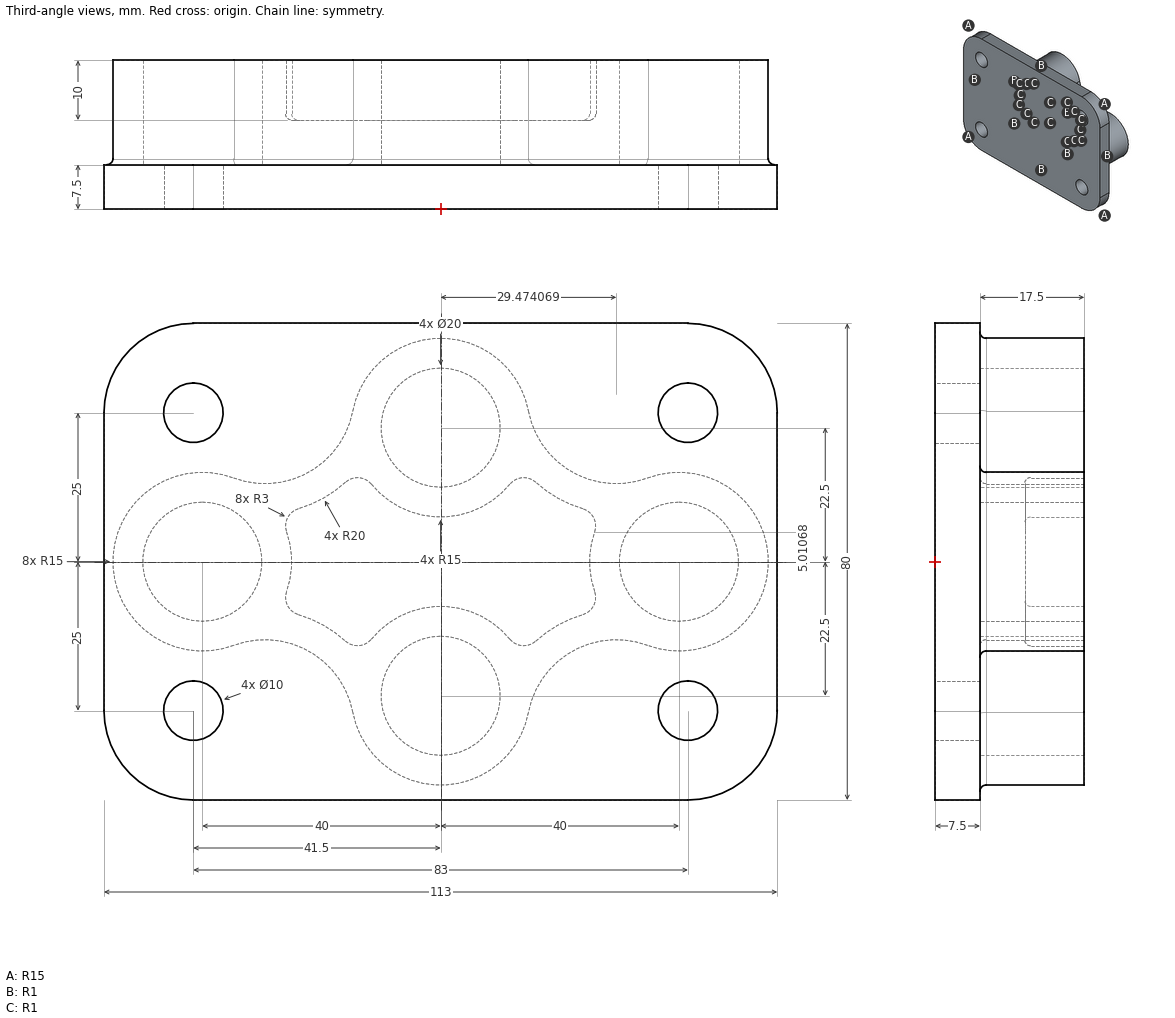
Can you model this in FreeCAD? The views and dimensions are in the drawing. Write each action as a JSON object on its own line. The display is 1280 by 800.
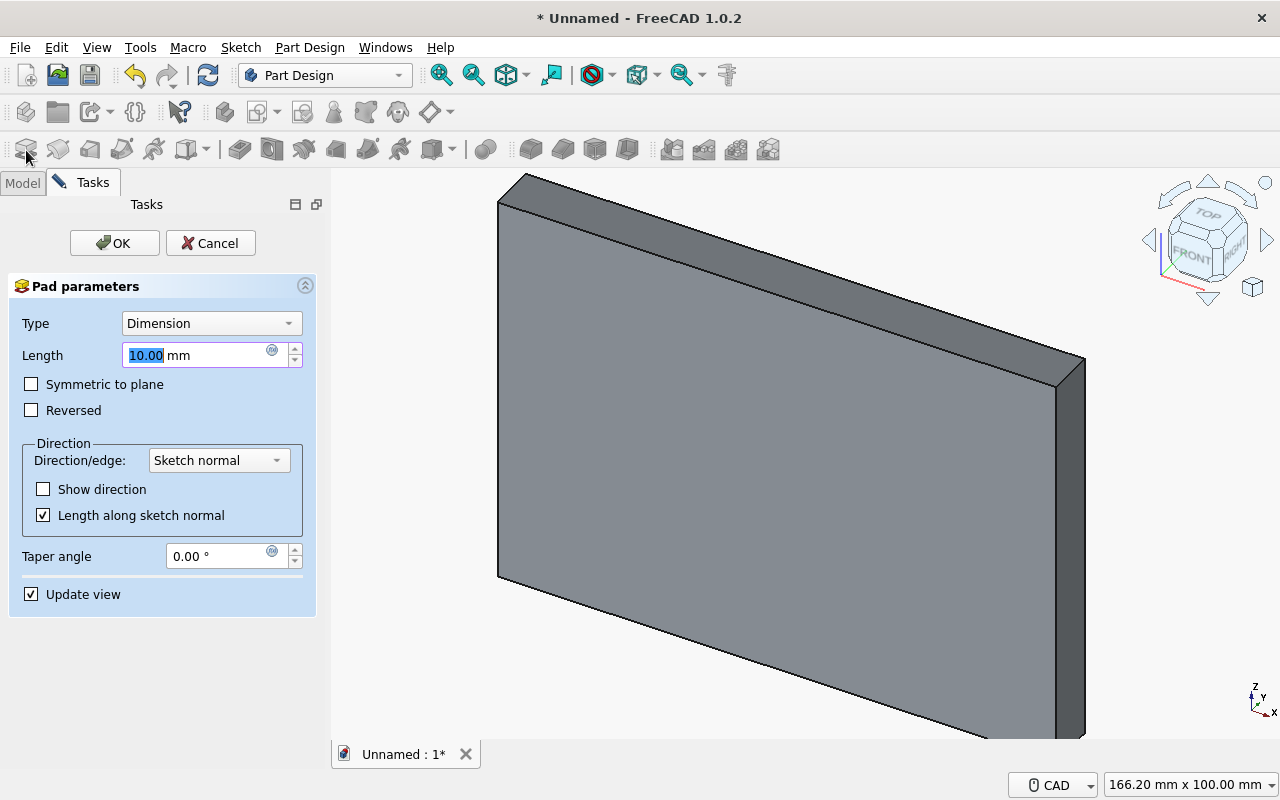
{"action": "type", "text": "7.5"}
{"action": "key", "text": "Tab"}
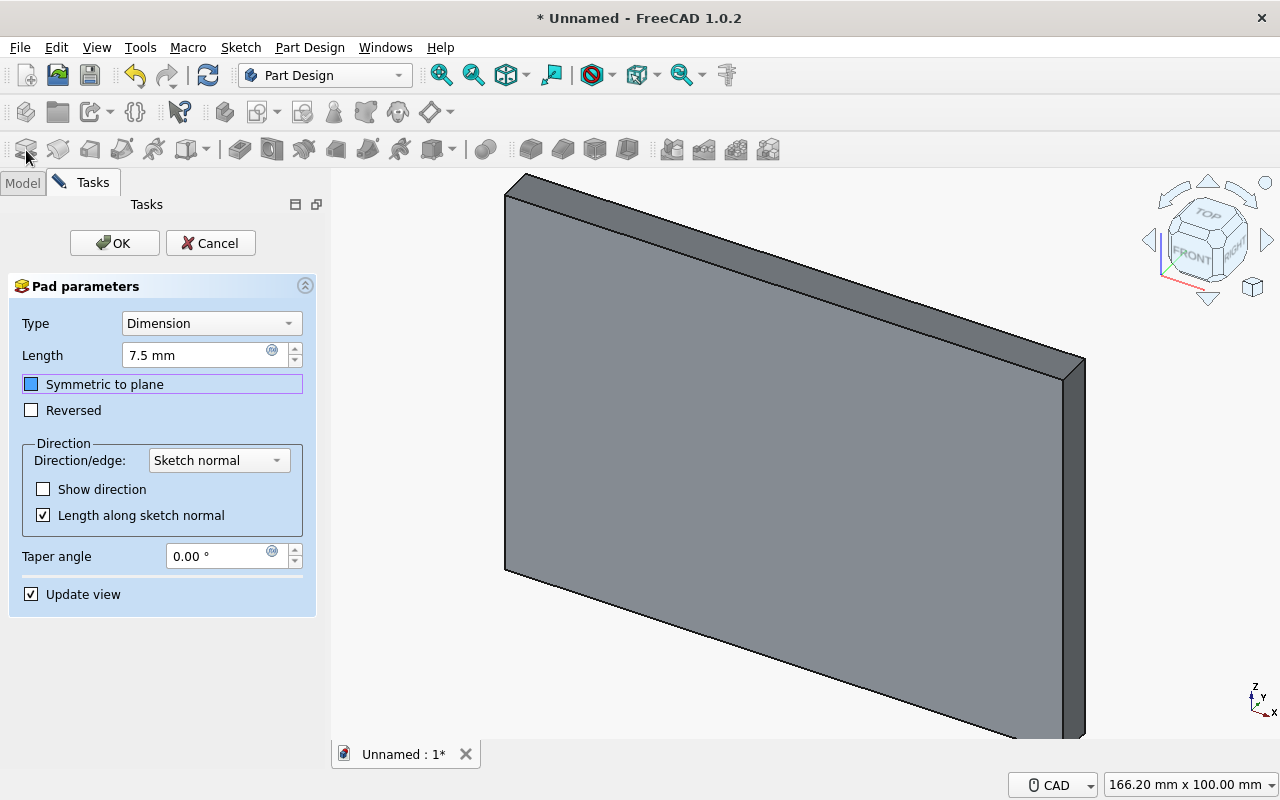
{"action": "left_click", "coordinate": [30, 410]}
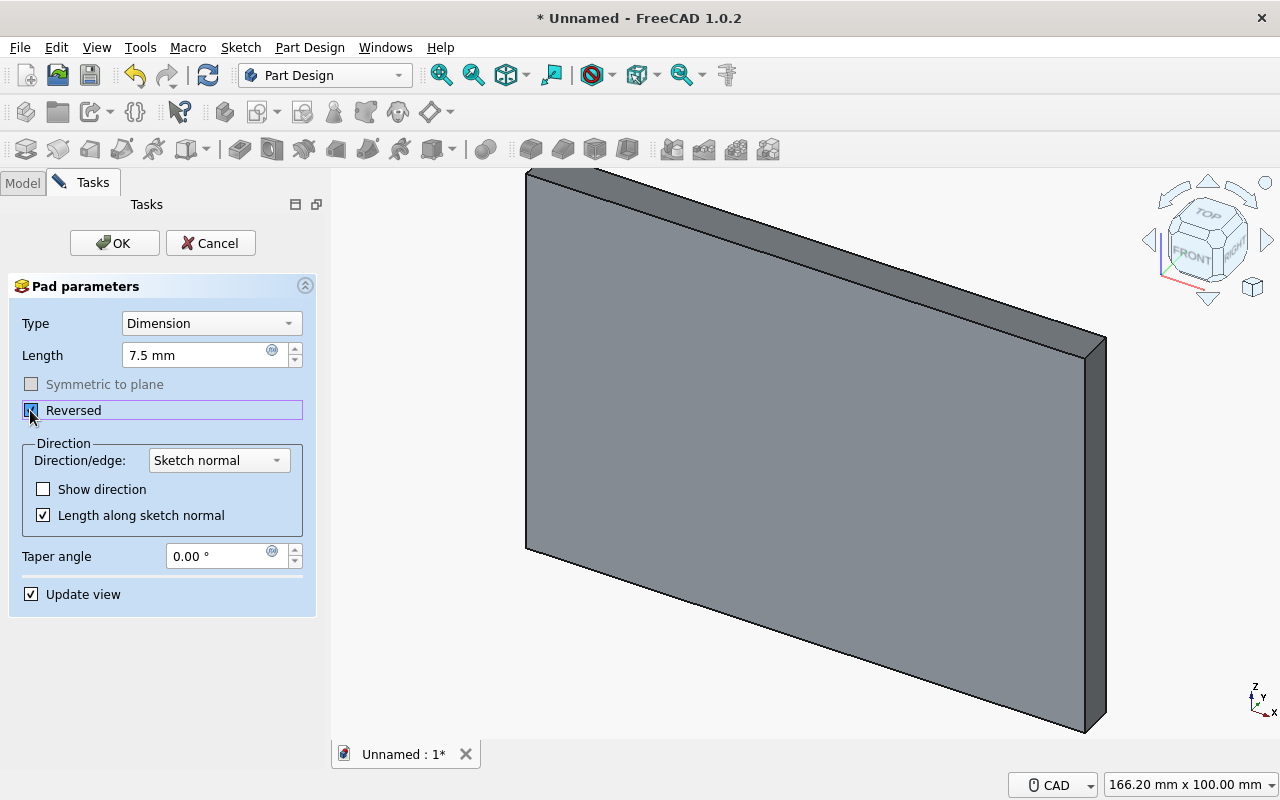
{"action": "left_click", "coordinate": [115, 243]}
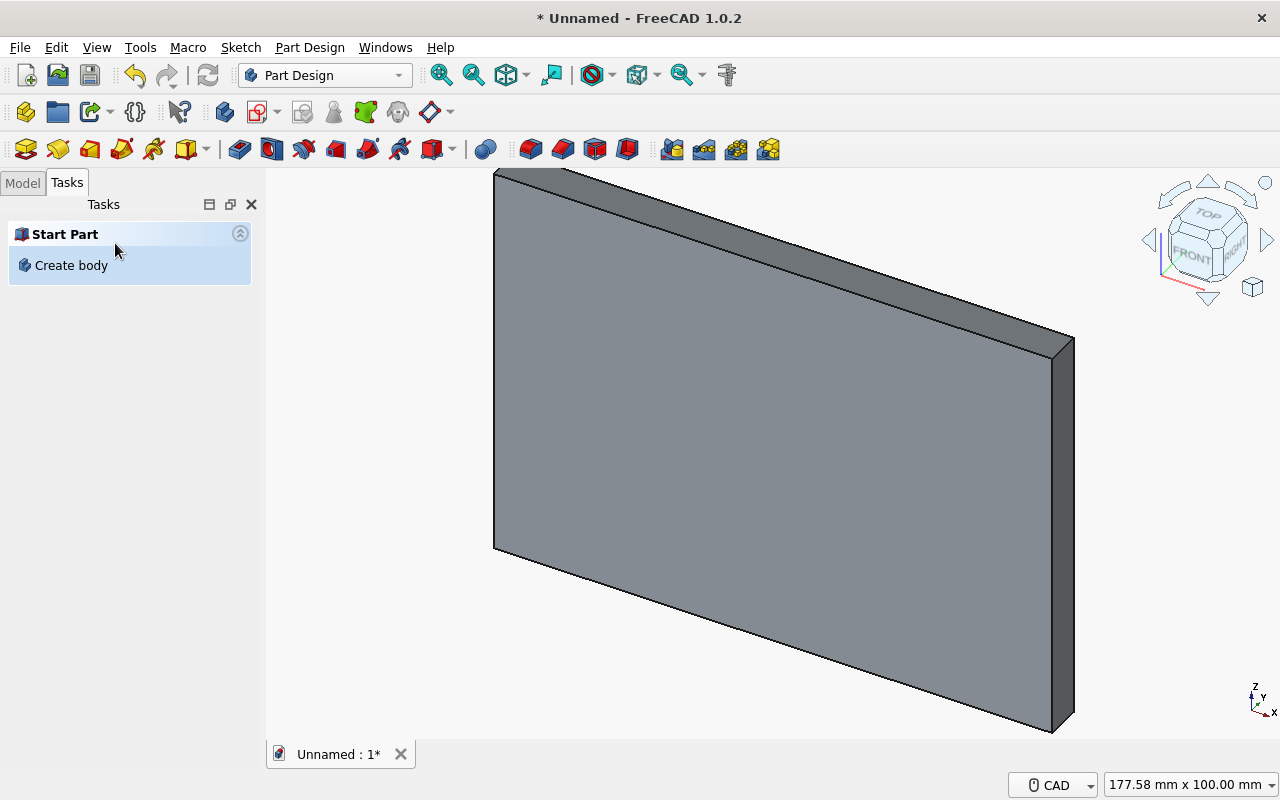
{"action": "left_click", "coordinate": [442, 76]}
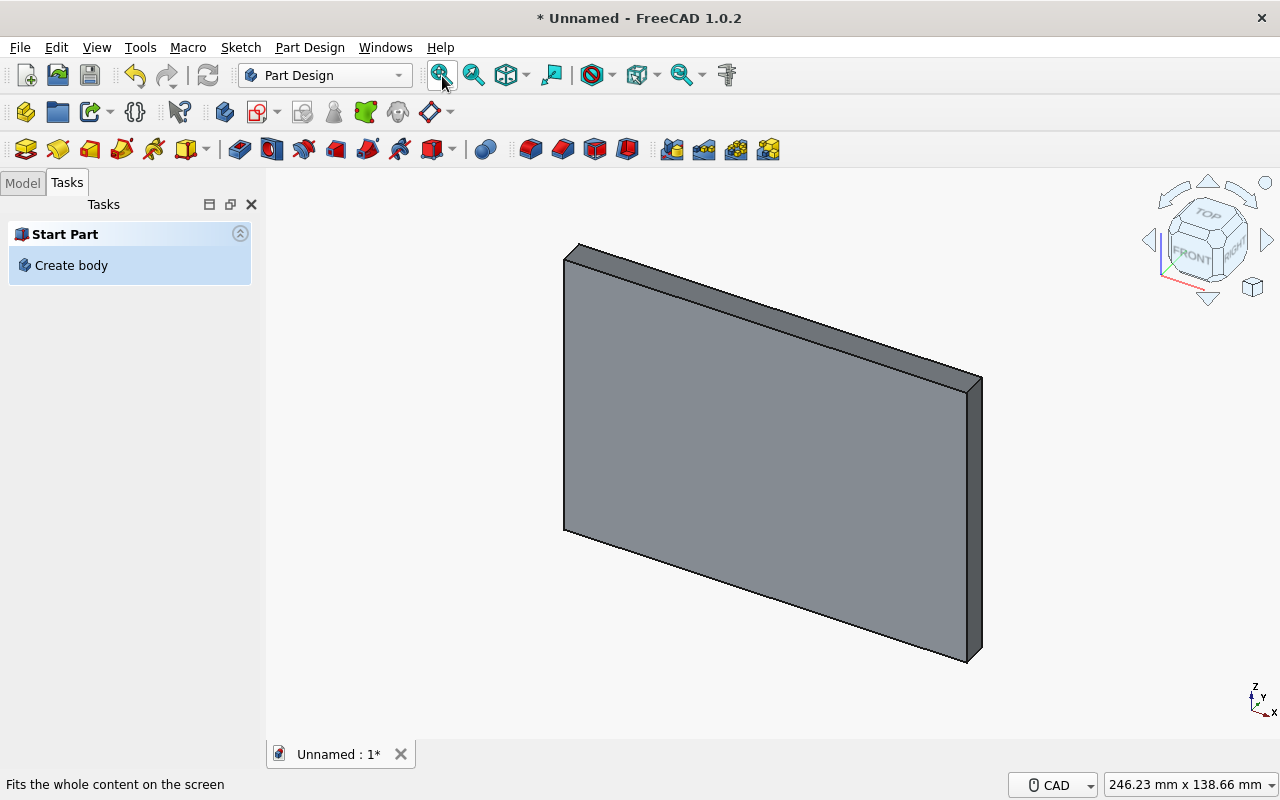
{"action": "left_click", "coordinate": [975, 384]}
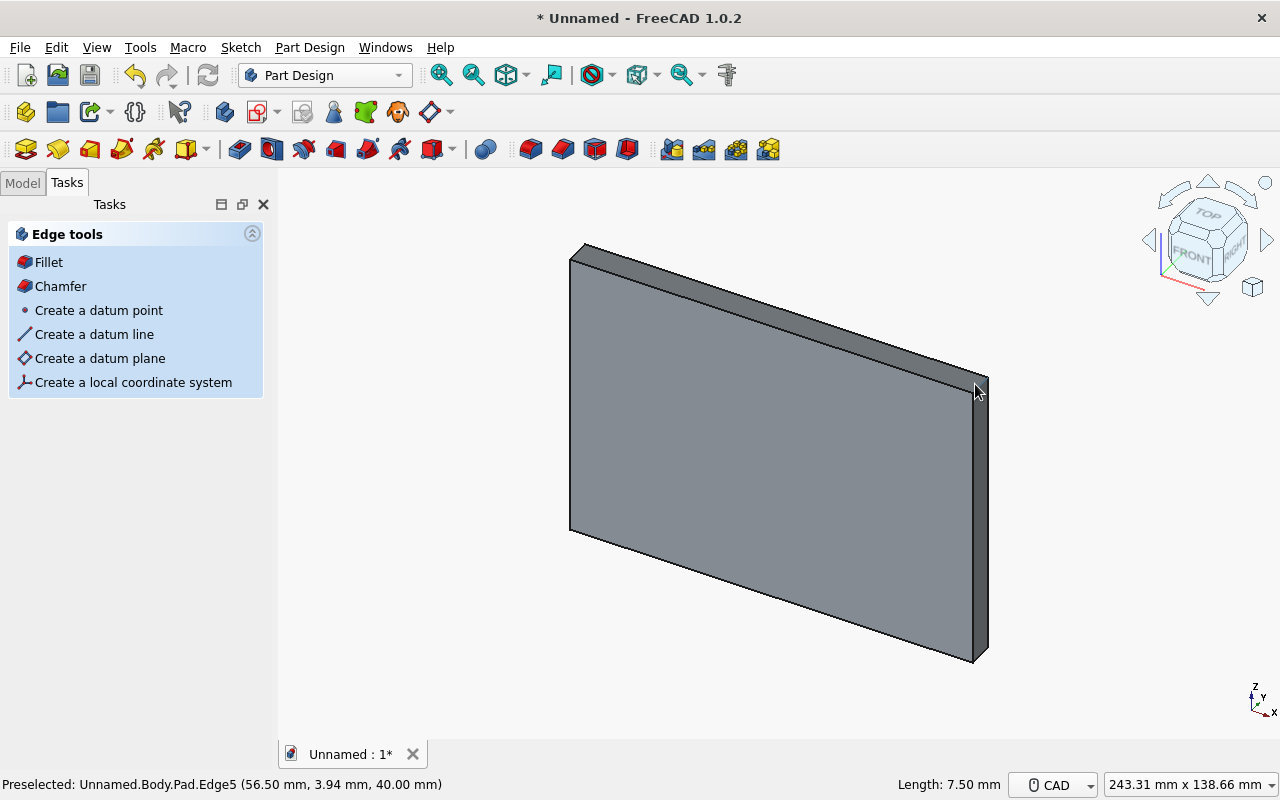
{"action": "key", "text": "0"}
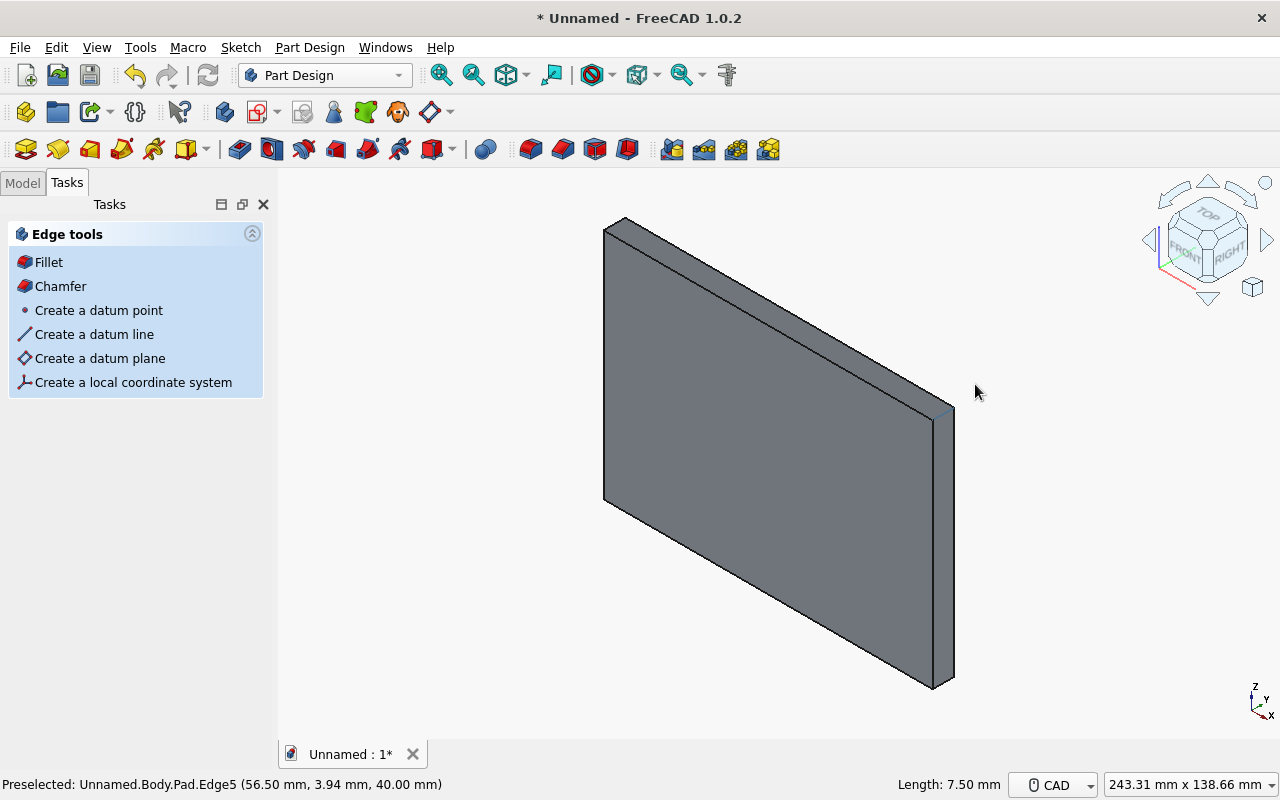
{"action": "key", "text": "2"}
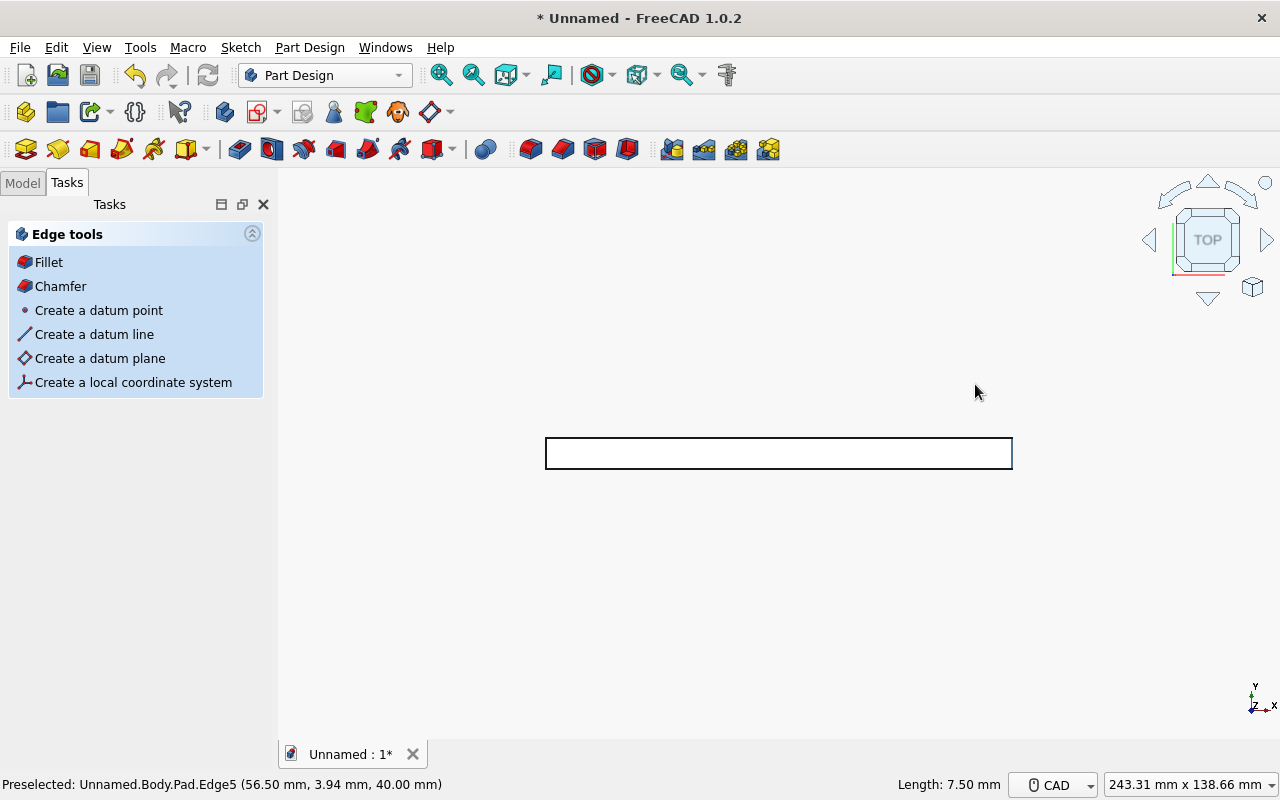
{"action": "left_click", "coordinate": [546, 453], "text": "ctrl"}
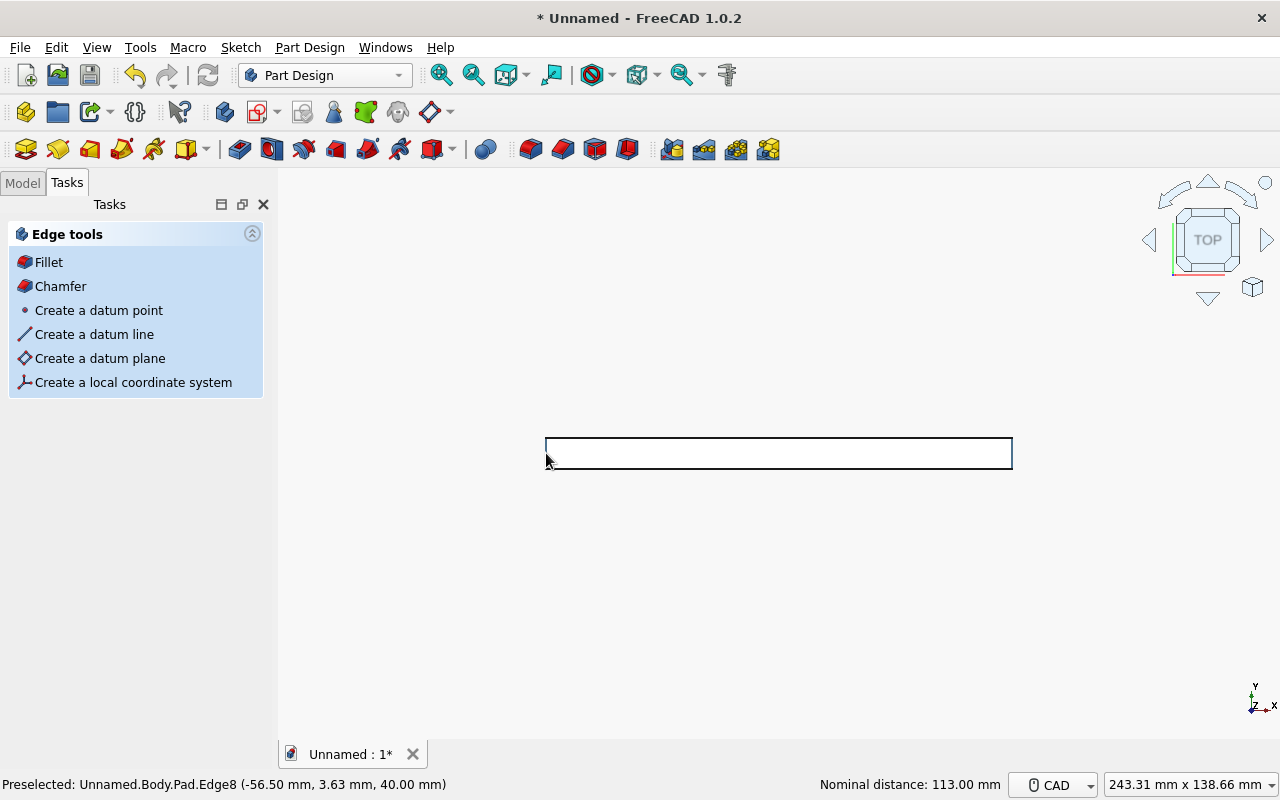
{"action": "key", "text": "1"}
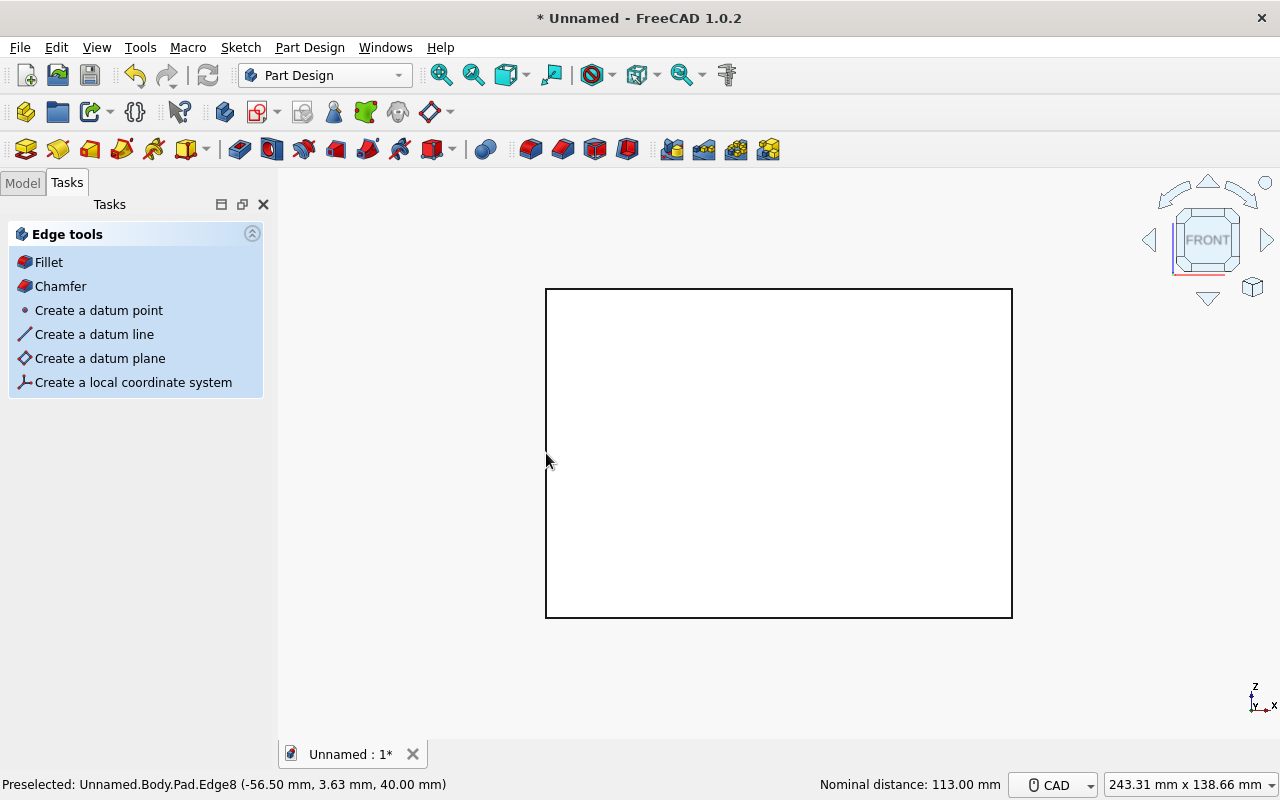
{"action": "key", "text": "3"}